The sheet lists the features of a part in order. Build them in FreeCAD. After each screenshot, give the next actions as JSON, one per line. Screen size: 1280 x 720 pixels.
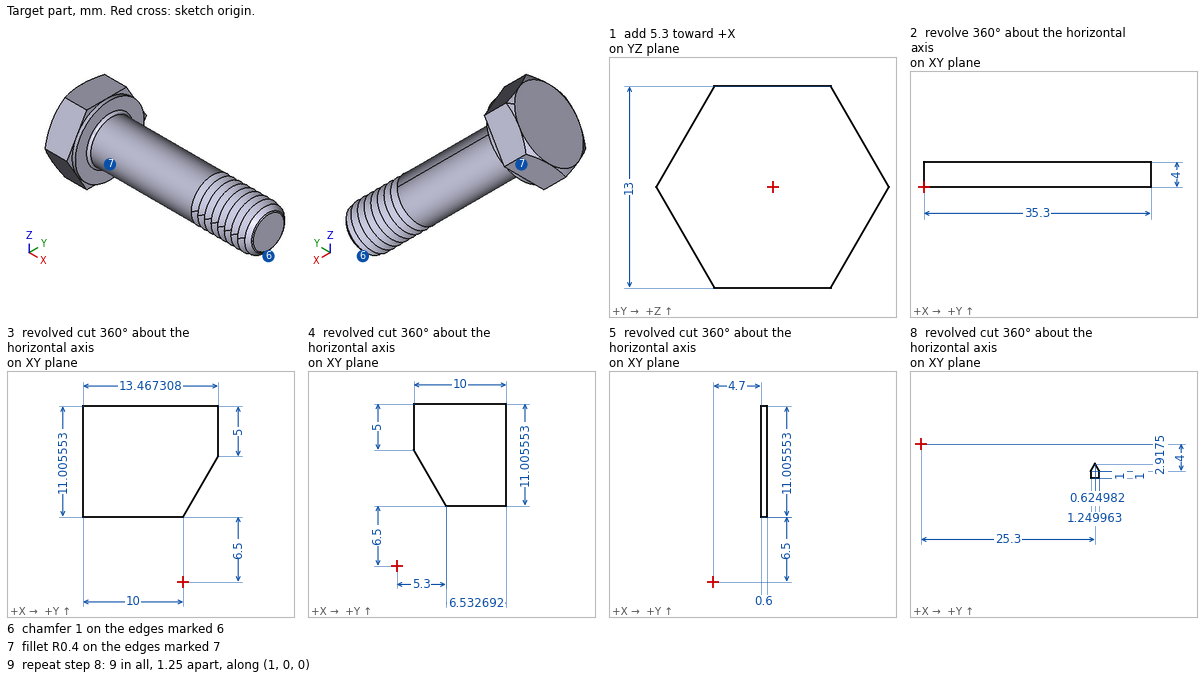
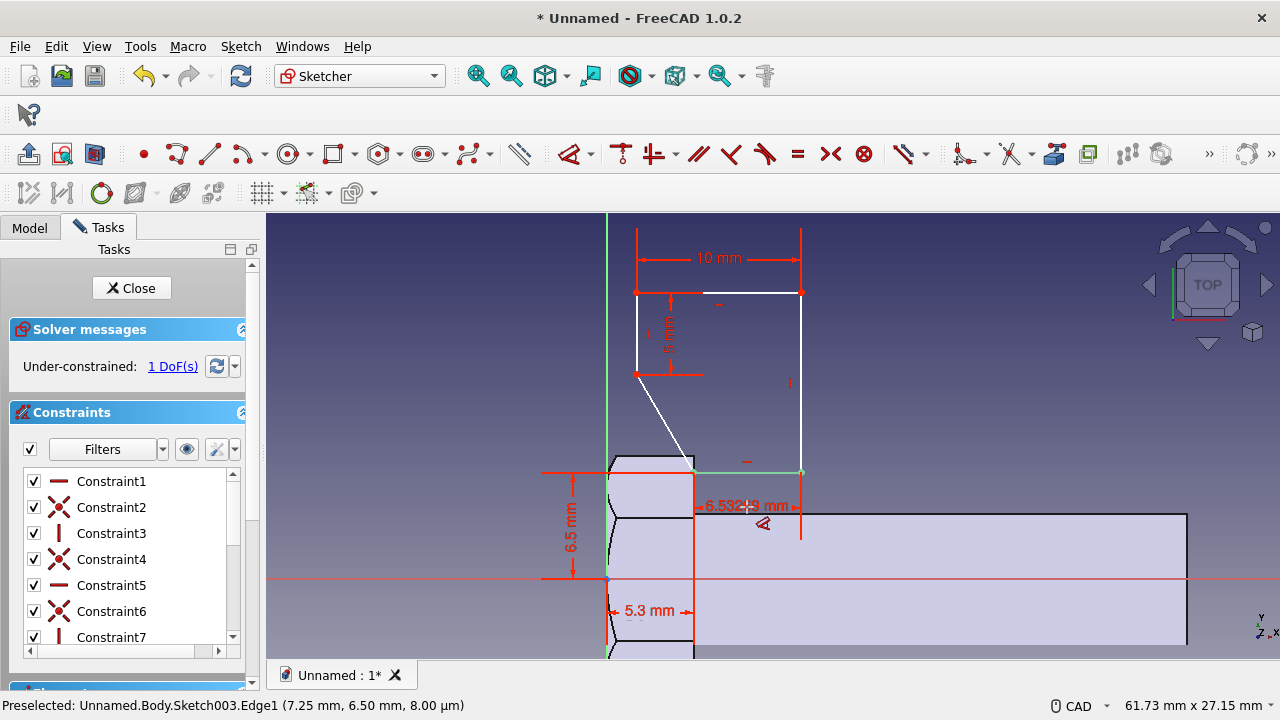
{"action": "left_click", "coordinate": [801, 419]}
{"action": "left_click", "coordinate": [835, 383]}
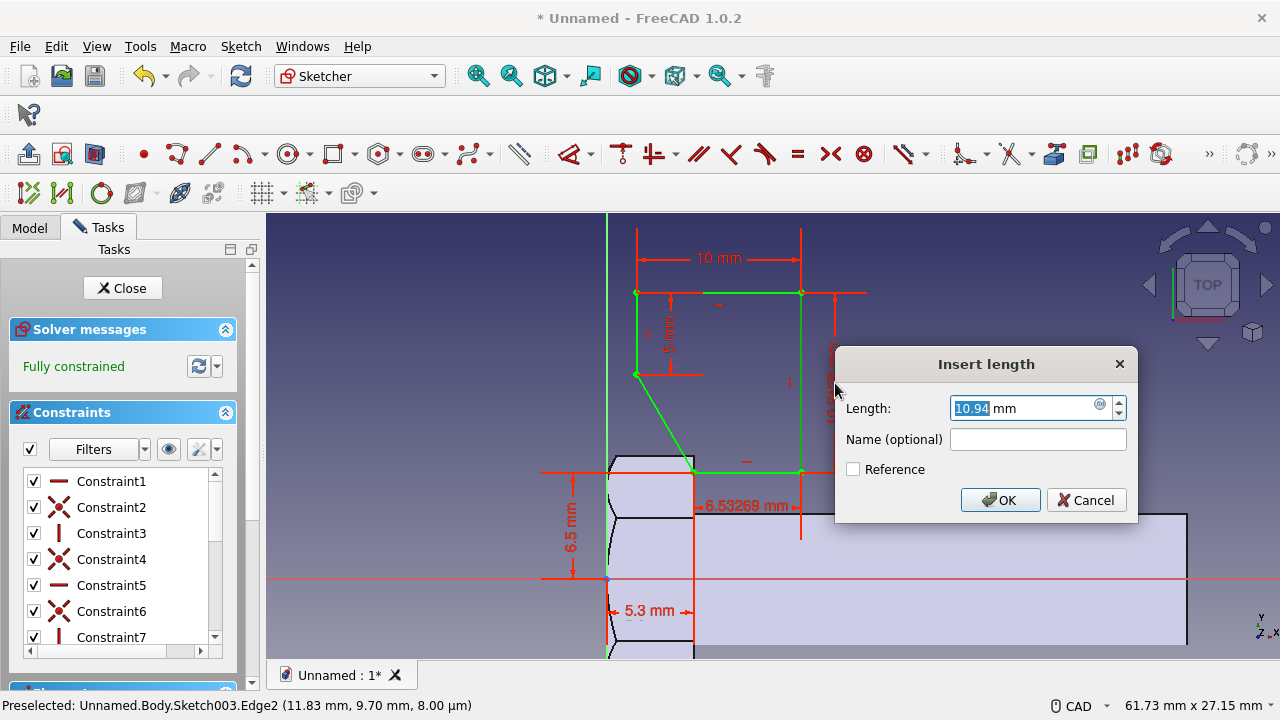
{"action": "type", "text": "11.005553"}
{"action": "key", "text": "Return"}
{"action": "key", "text": "Escape"}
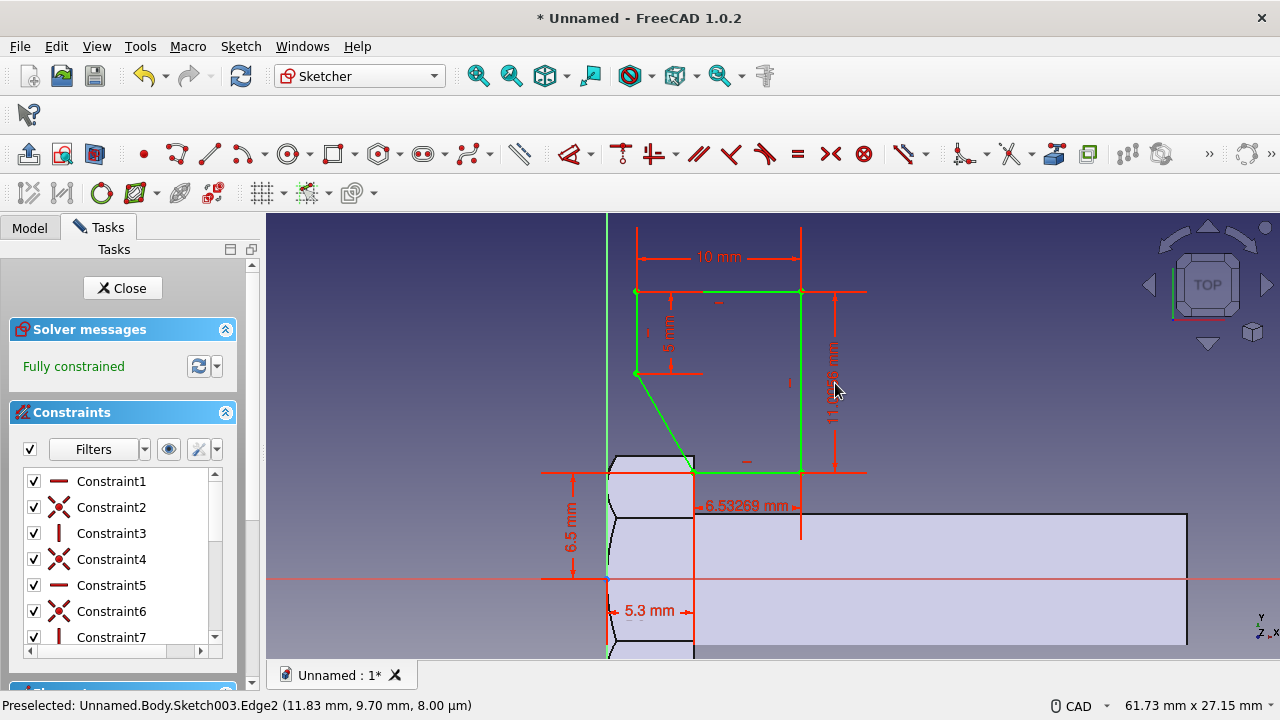
{"action": "left_click", "coordinate": [123, 288]}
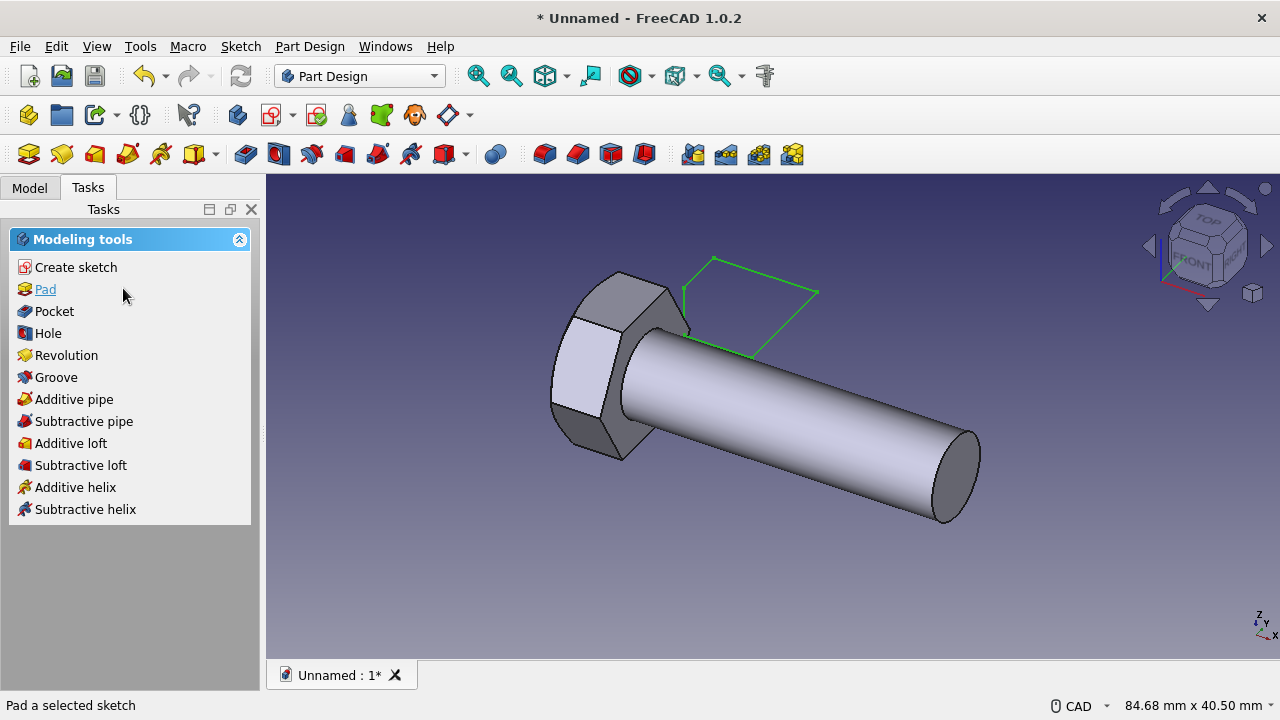
{"action": "left_click", "coordinate": [312, 154]}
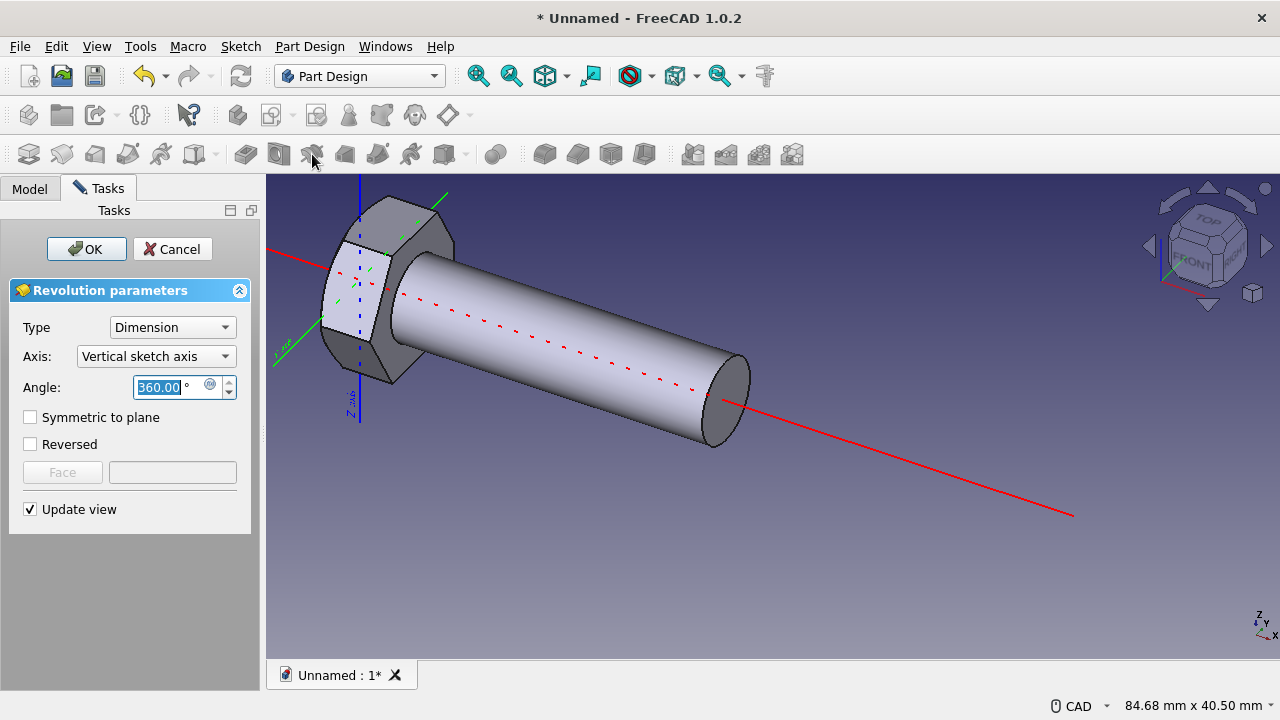
{"action": "left_click", "coordinate": [157, 356]}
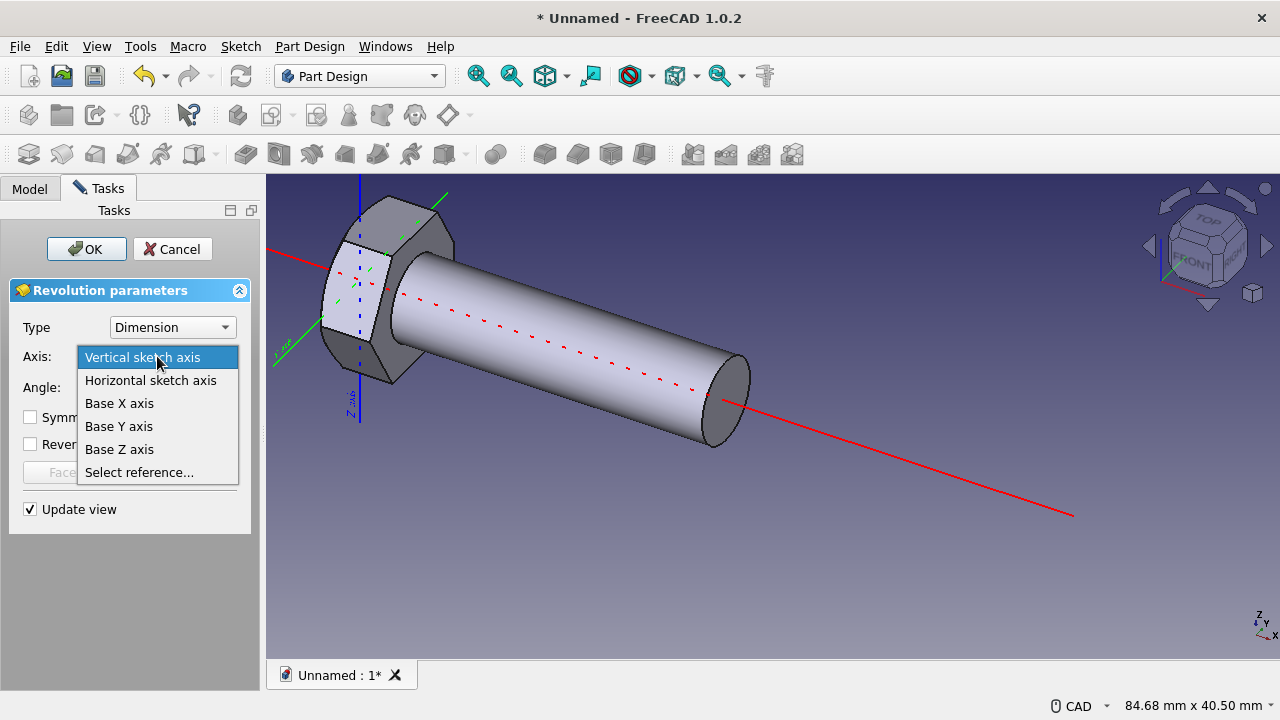
{"action": "left_click", "coordinate": [156, 380]}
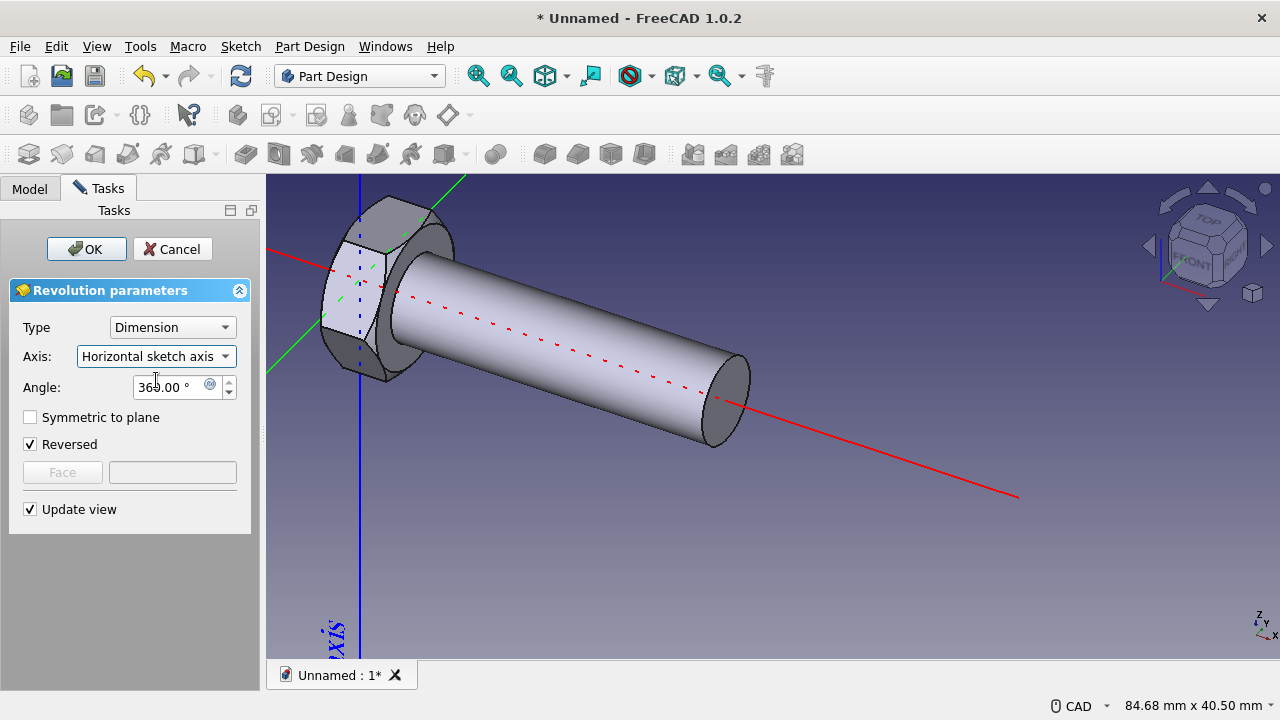
{"action": "left_click", "coordinate": [87, 249]}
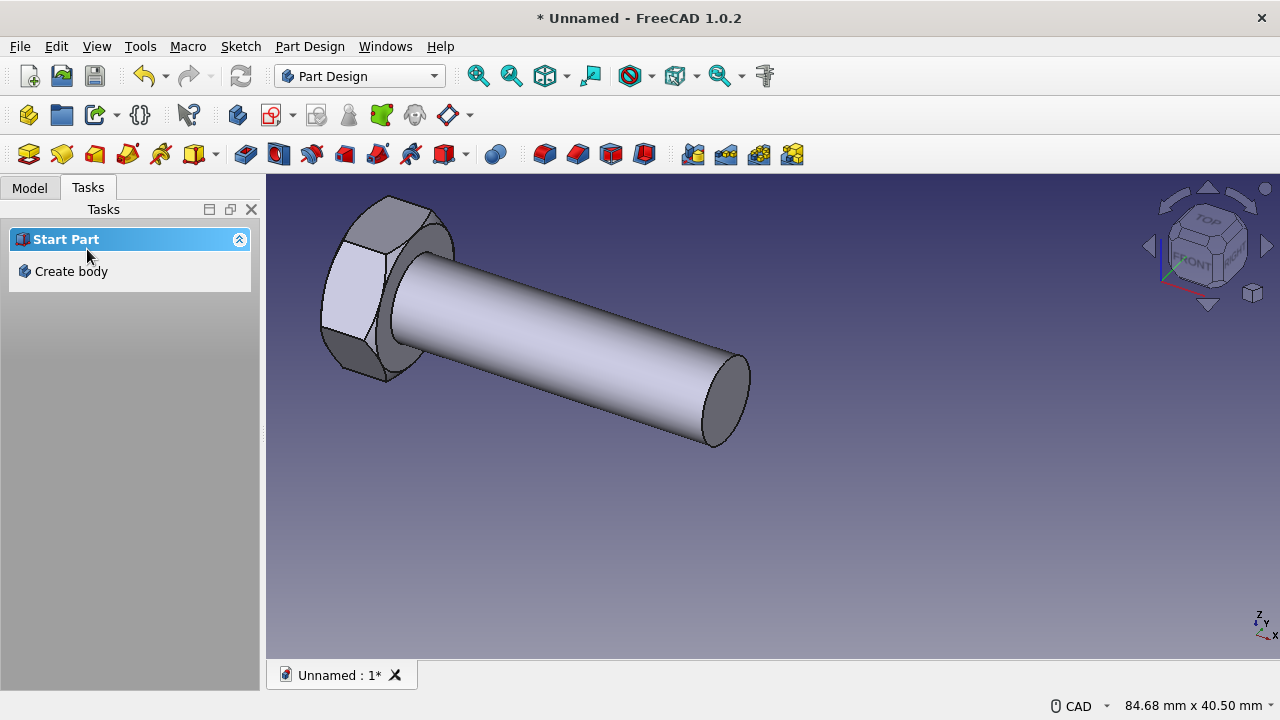
{"action": "left_click", "coordinate": [479, 76]}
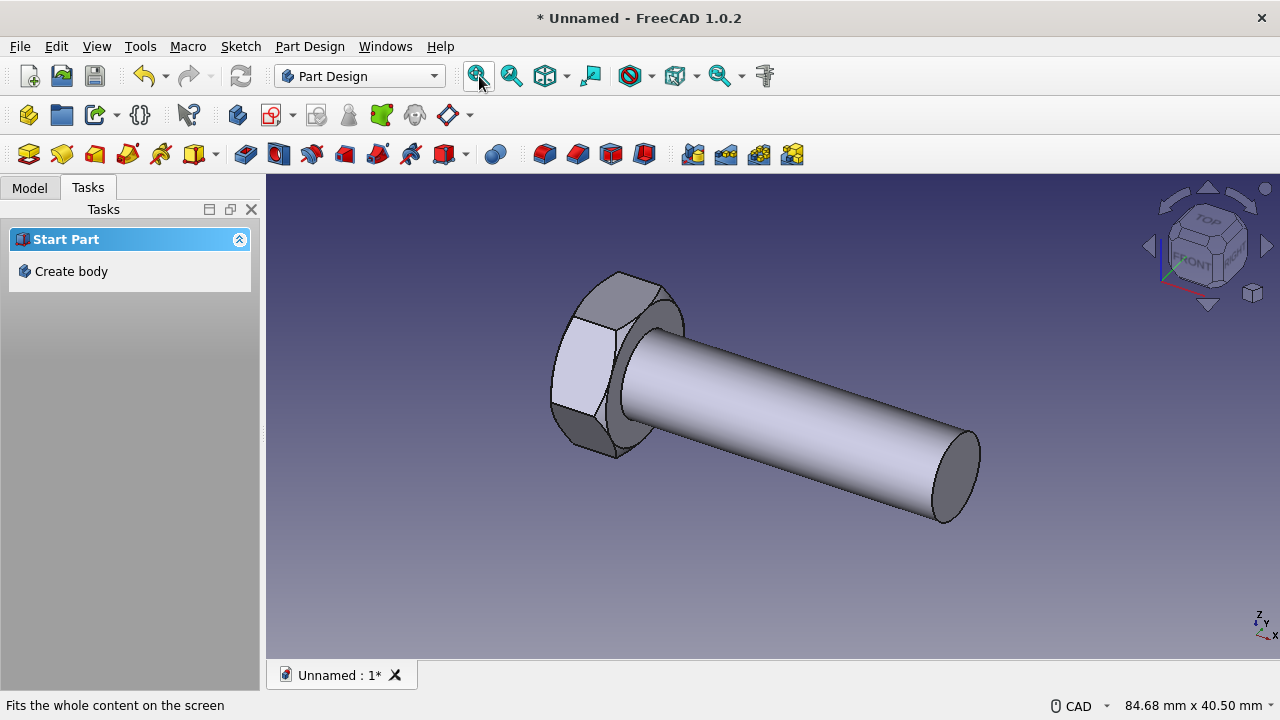
{"action": "left_click", "coordinate": [270, 116]}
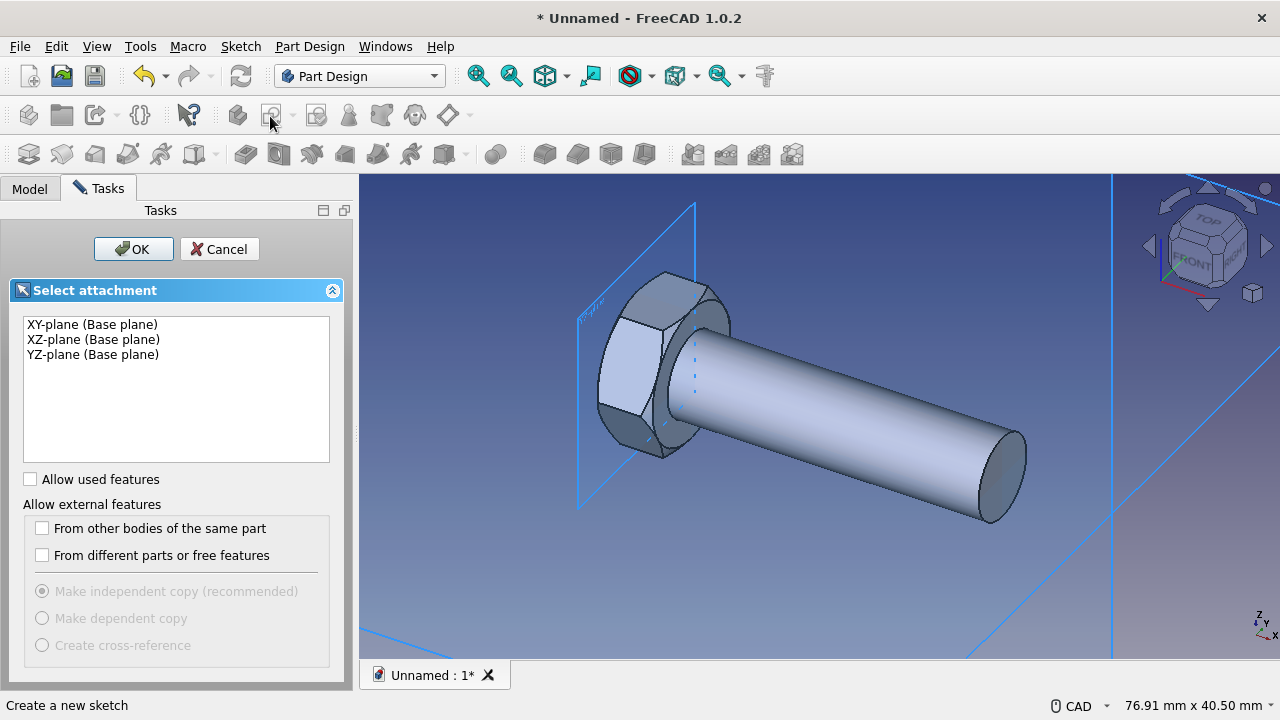
{"action": "left_click", "coordinate": [84, 324]}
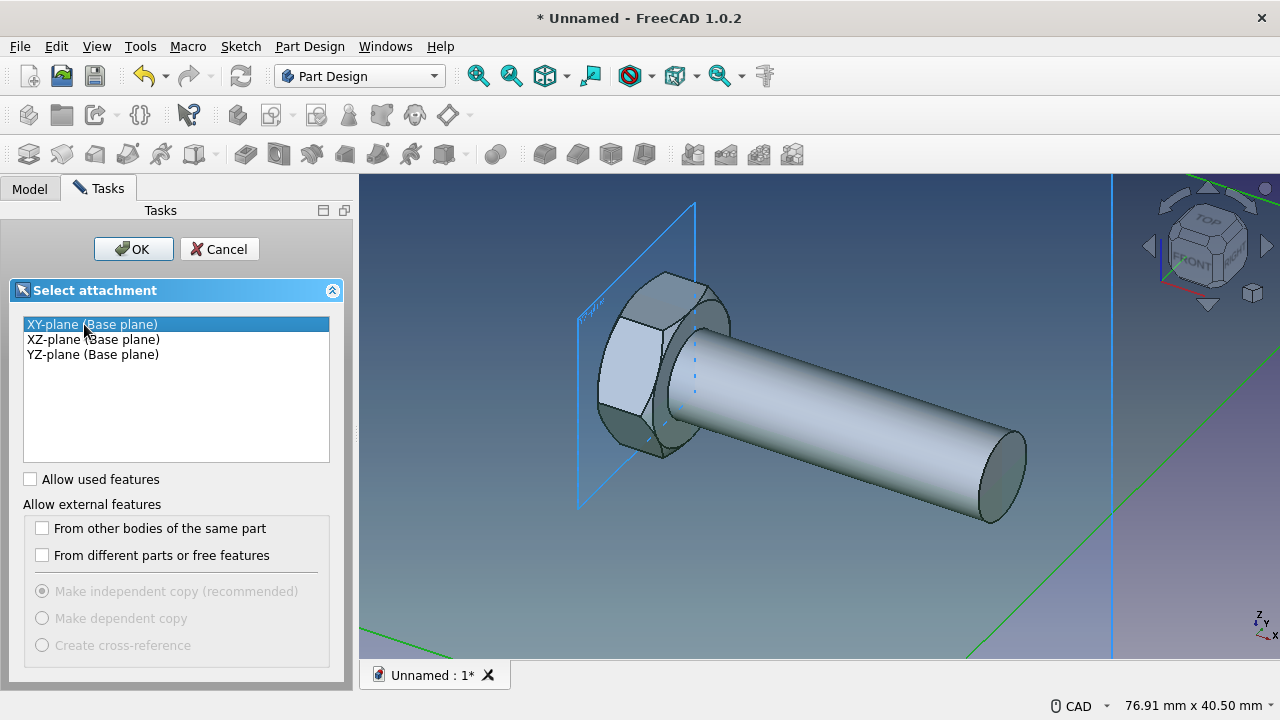
{"action": "left_click", "coordinate": [134, 249]}